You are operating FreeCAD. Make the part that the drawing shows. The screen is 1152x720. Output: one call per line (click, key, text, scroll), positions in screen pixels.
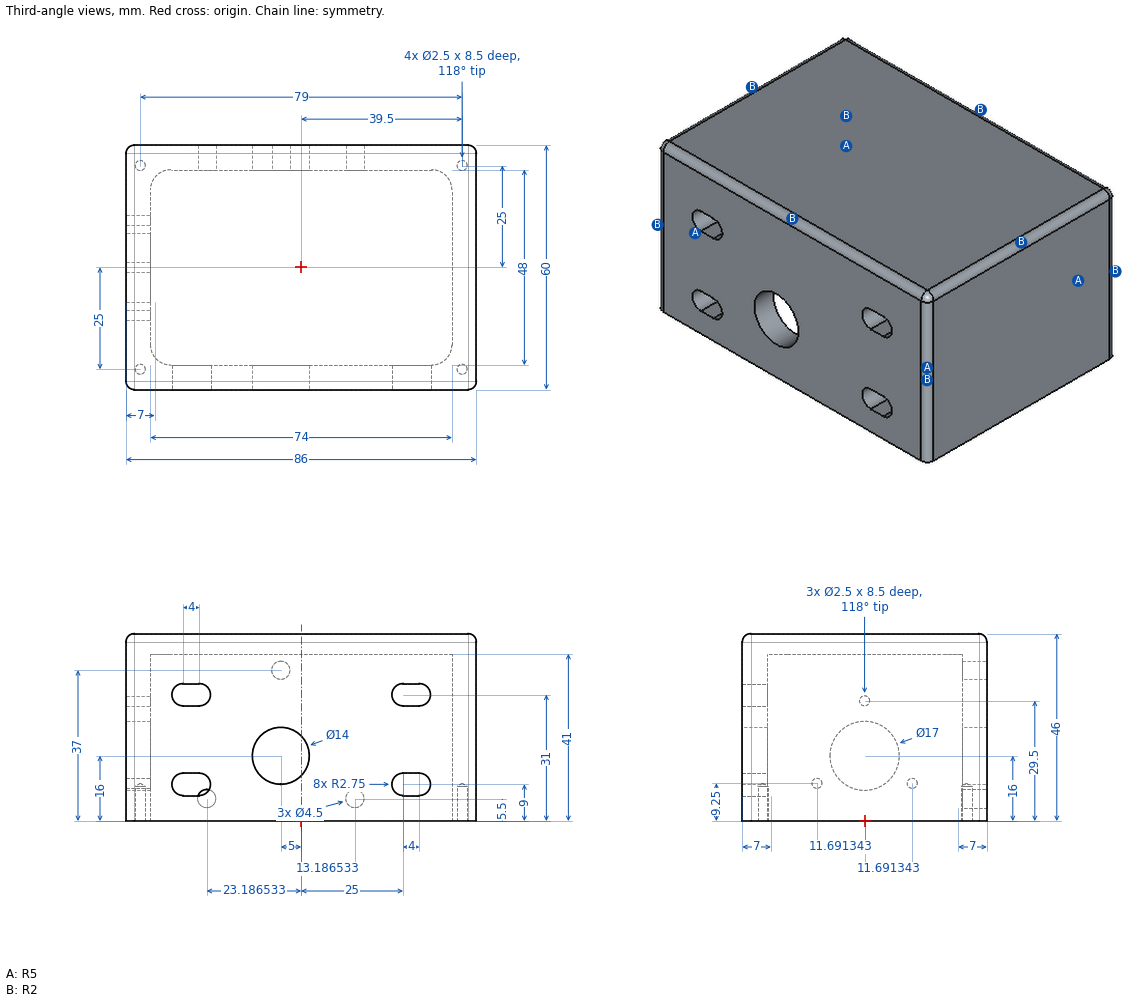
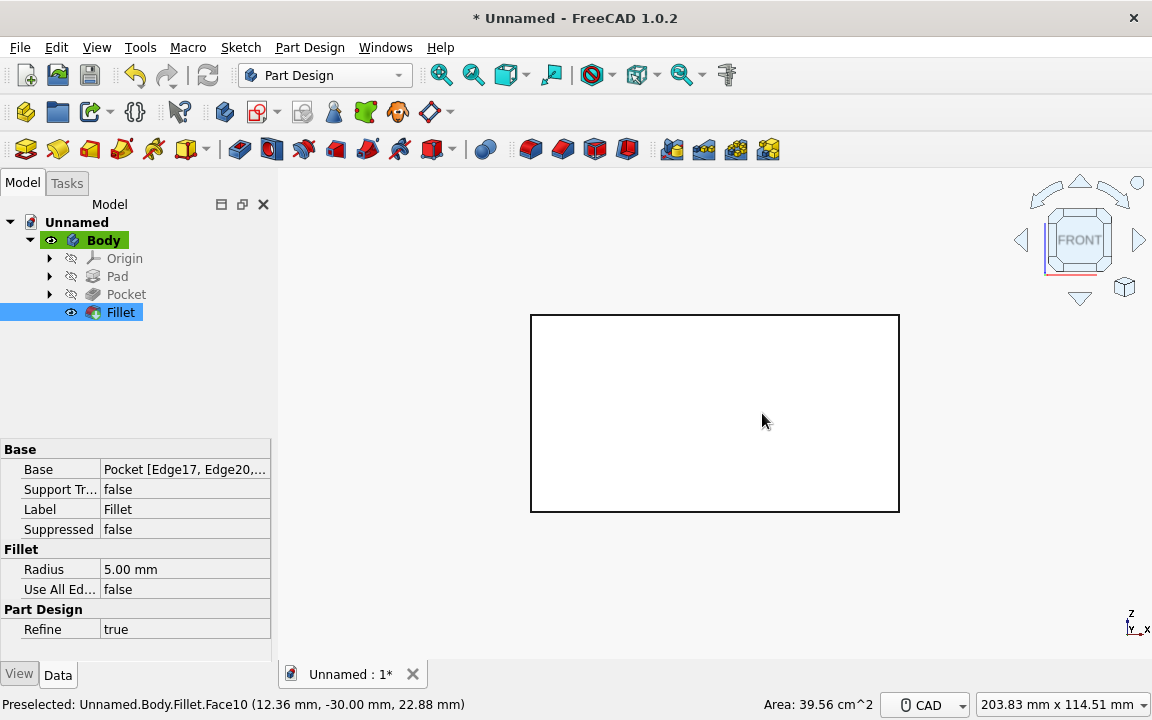
click(258, 112)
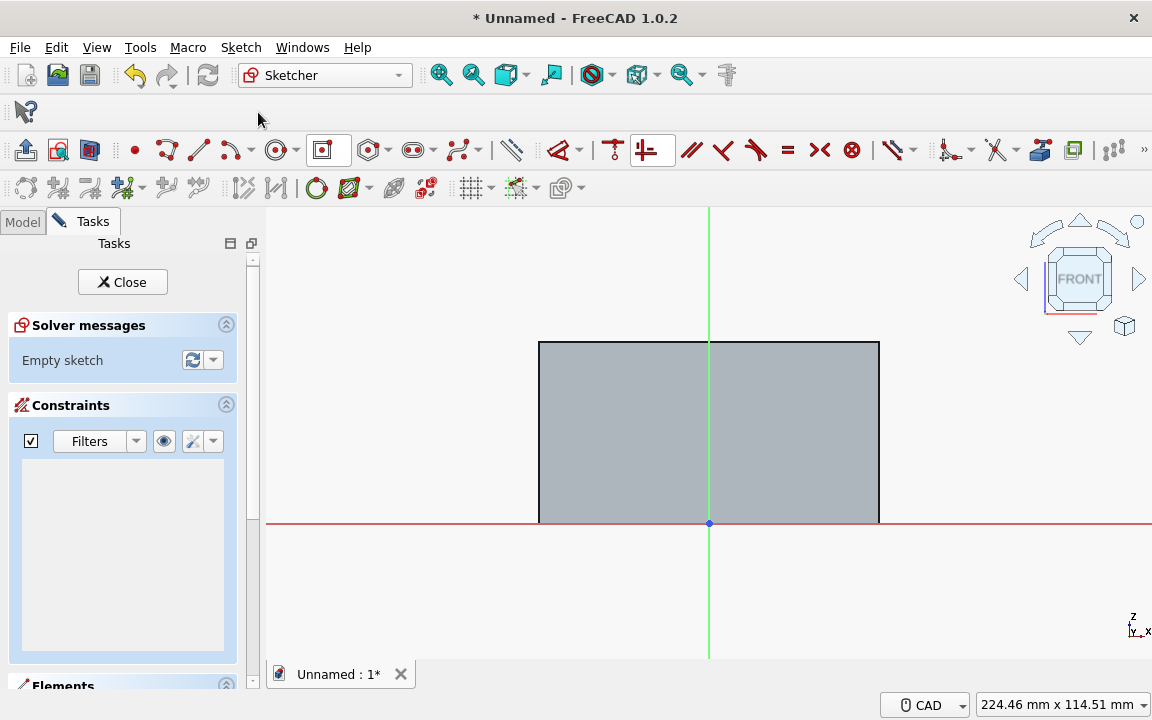
scroll(792, 487, up, 3)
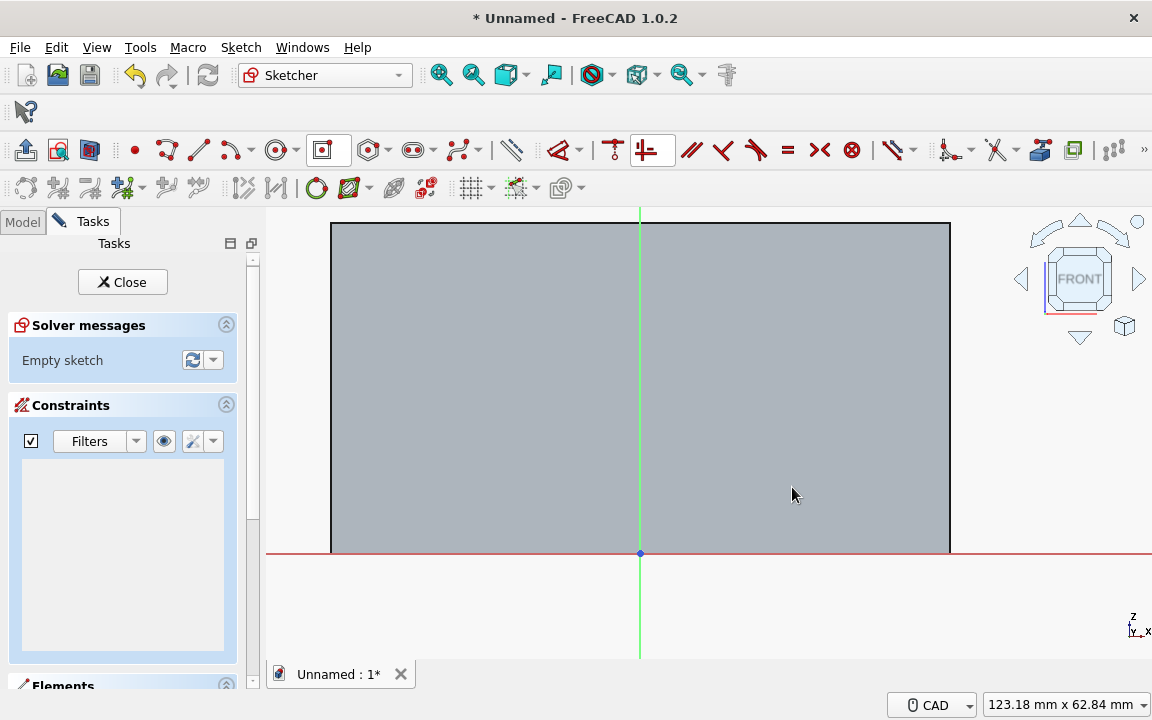
click(414, 150)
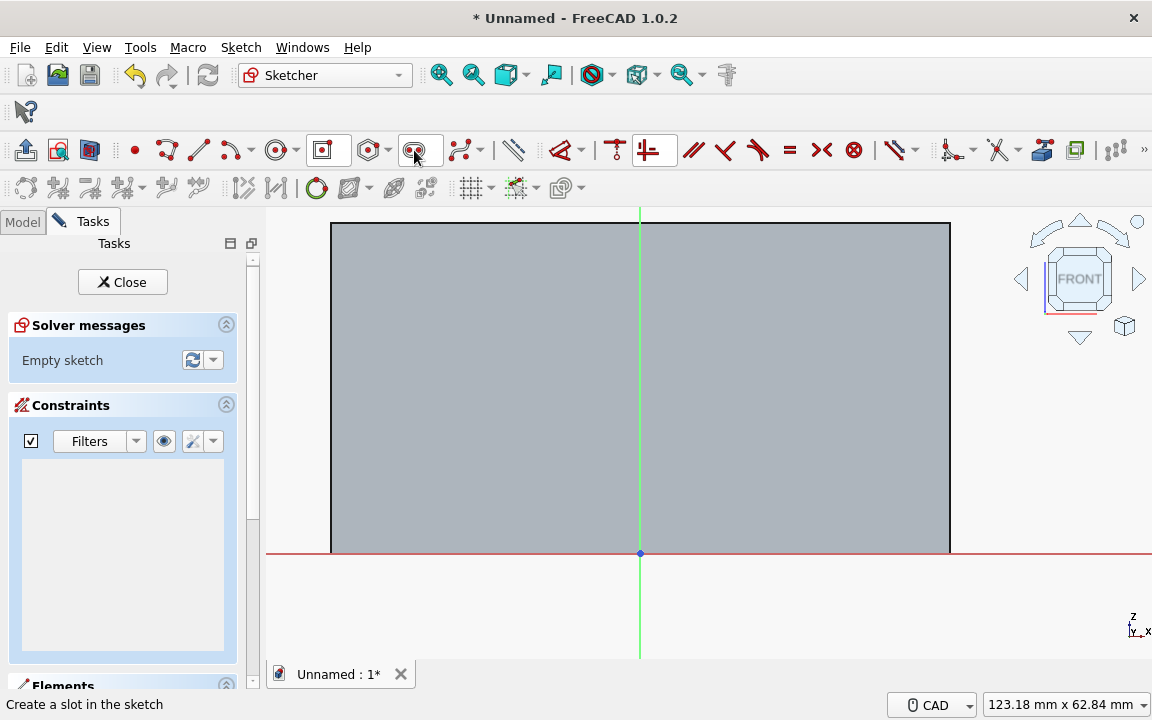
click(820, 489)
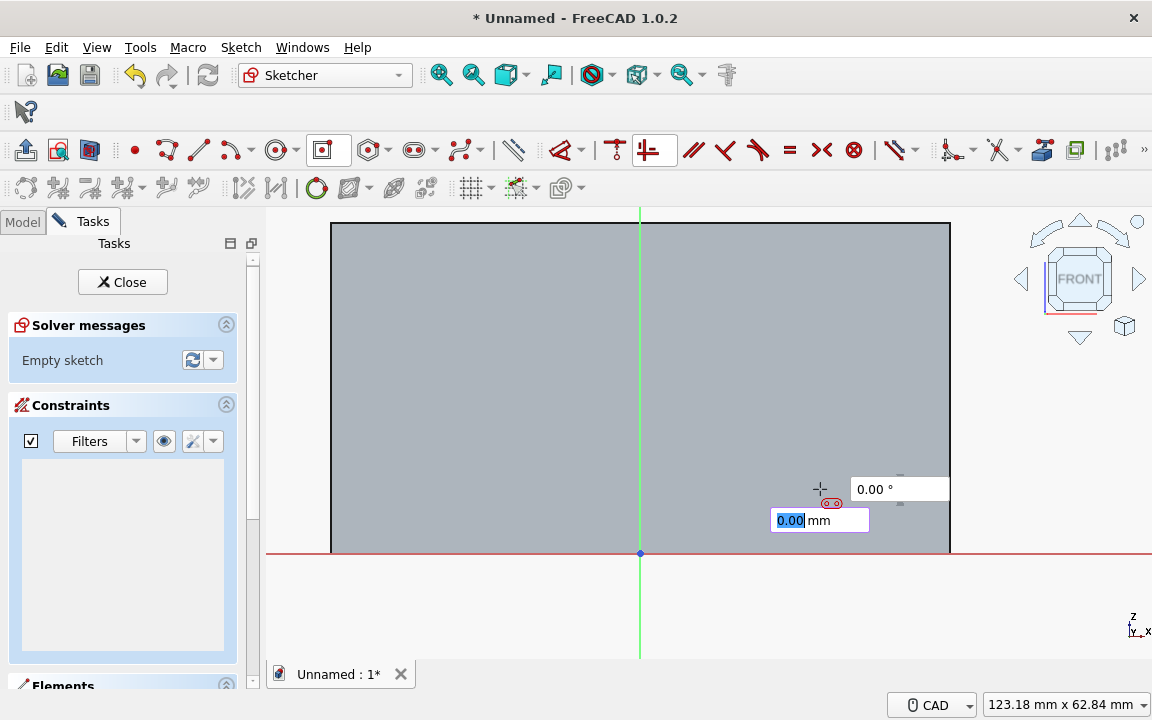
click(849, 489)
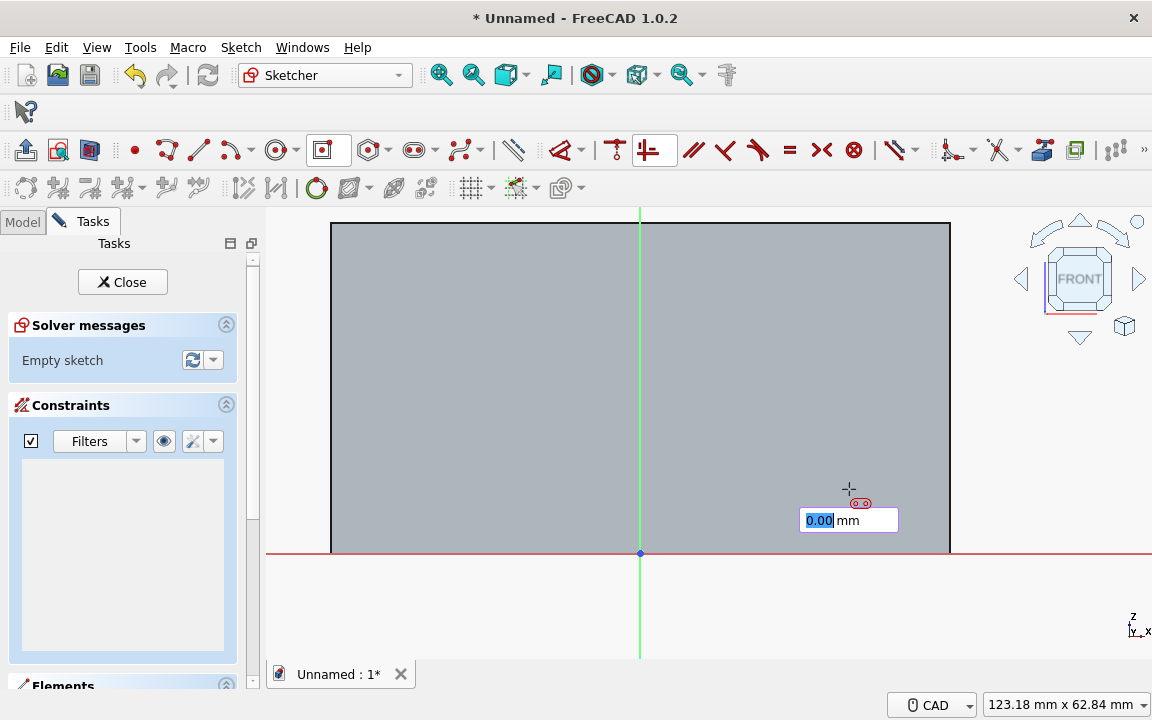
click(834, 469)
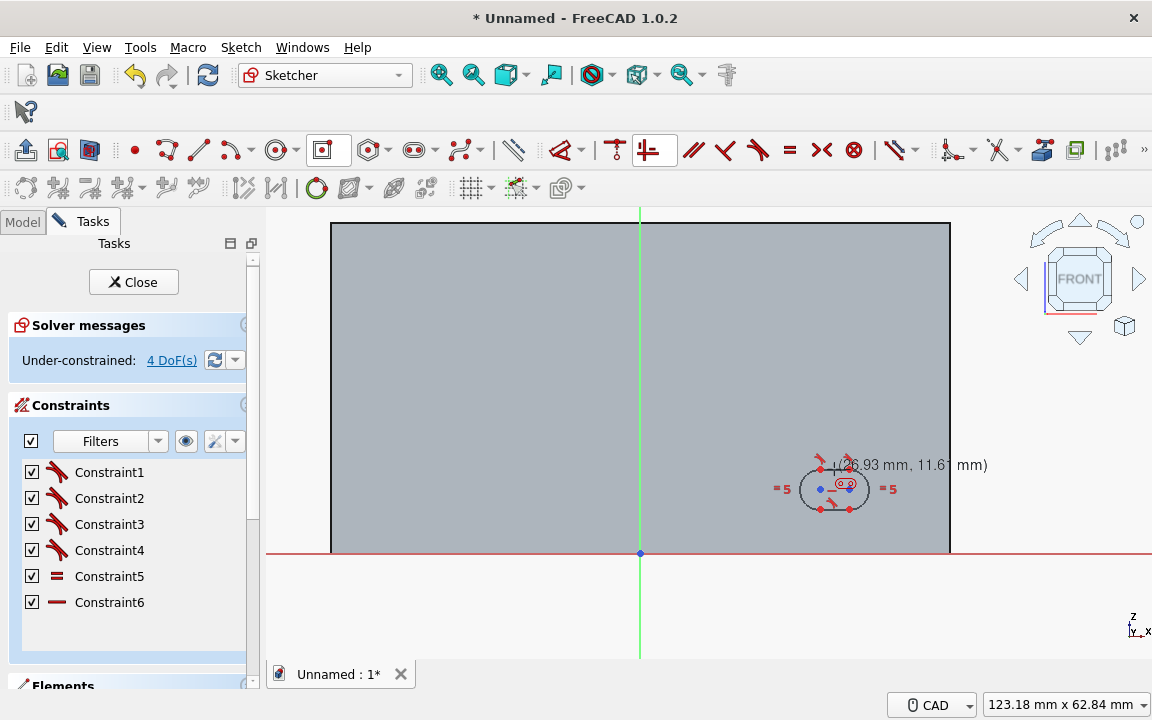
click(820, 331)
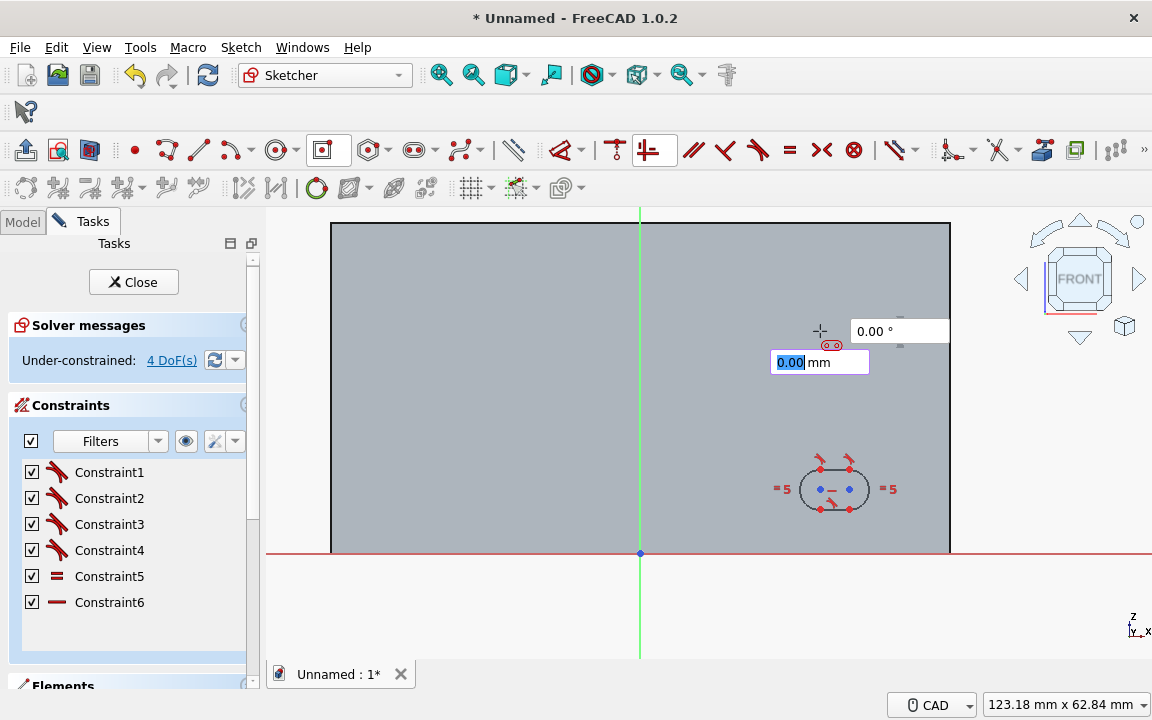
click(849, 331)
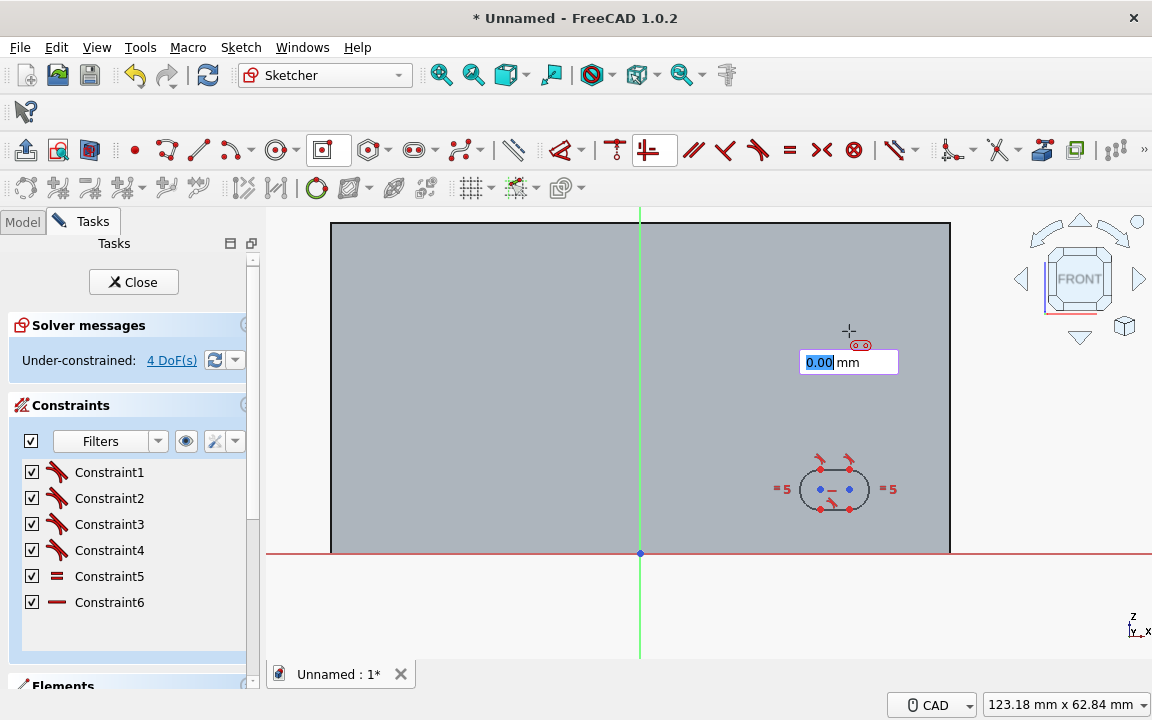
click(834, 311)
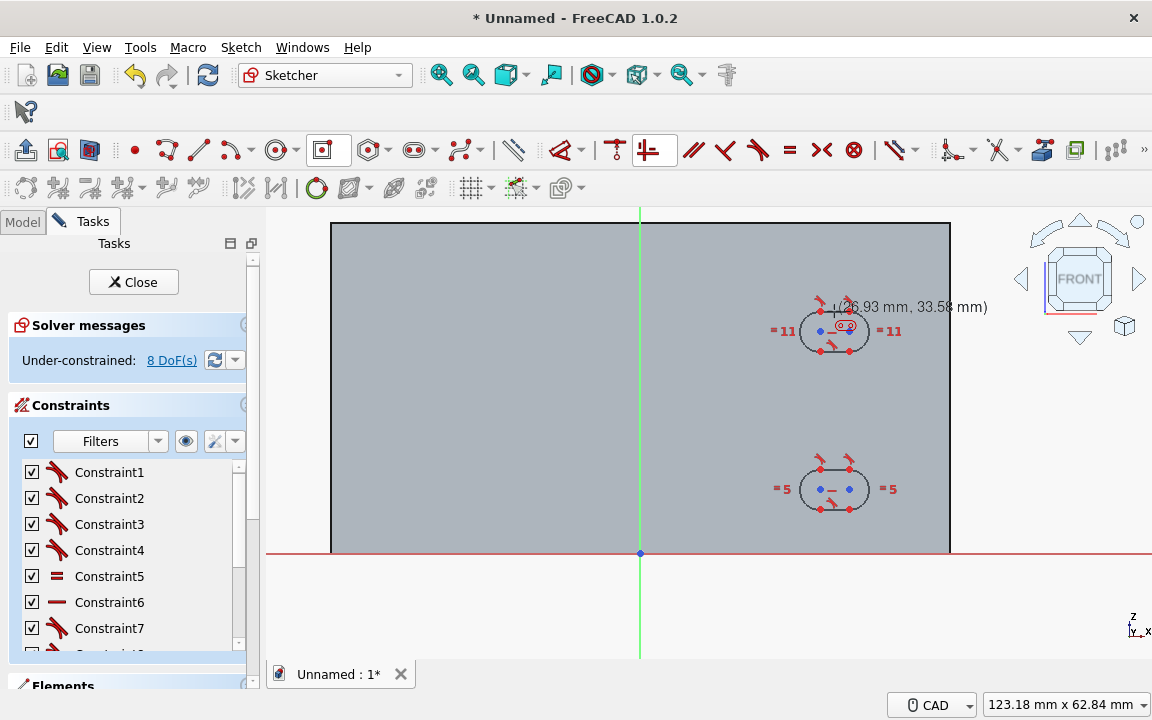
click(432, 331)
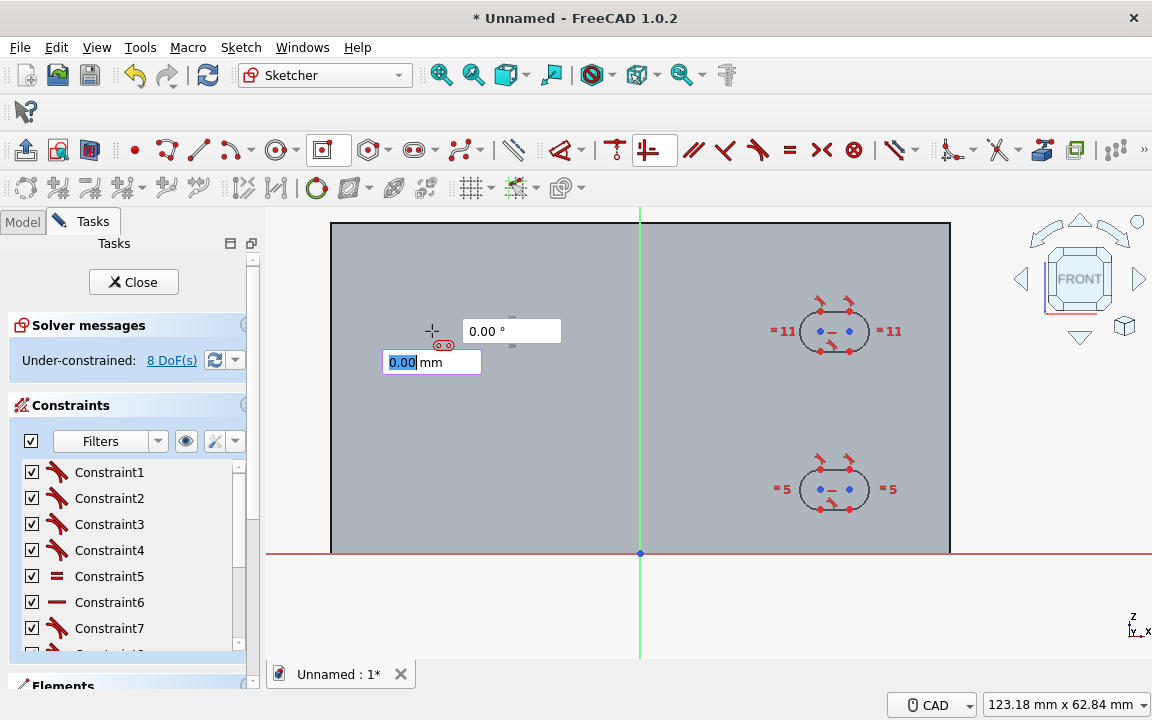
click(460, 331)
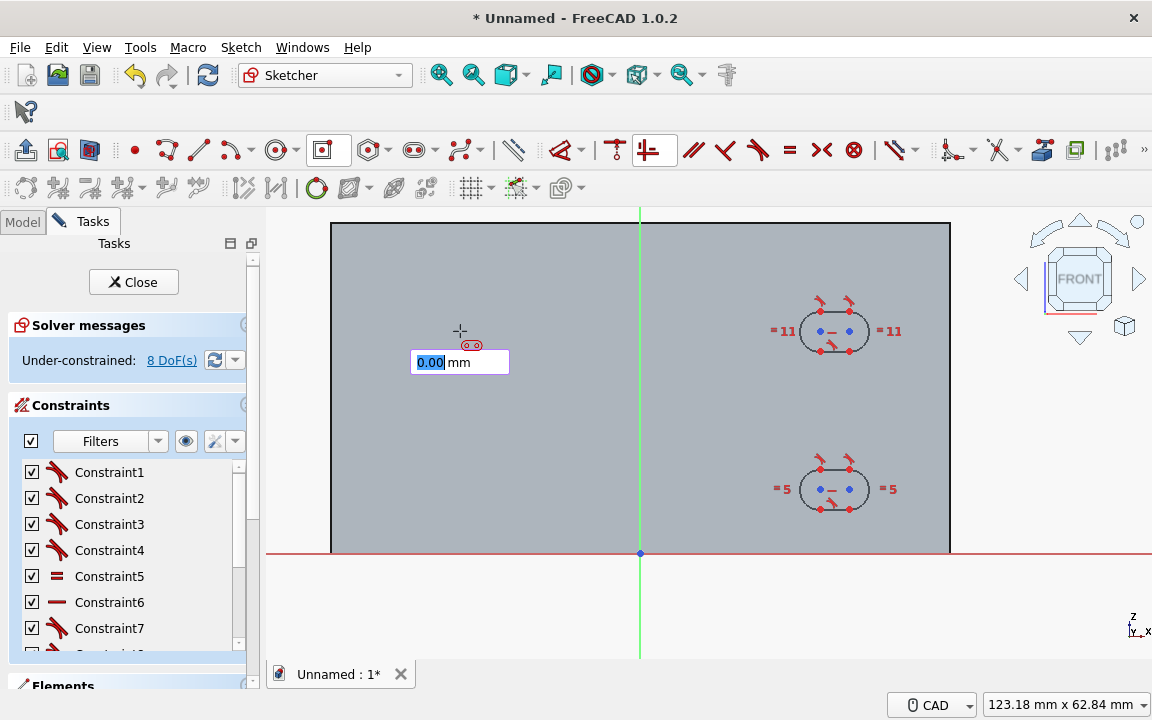
click(446, 311)